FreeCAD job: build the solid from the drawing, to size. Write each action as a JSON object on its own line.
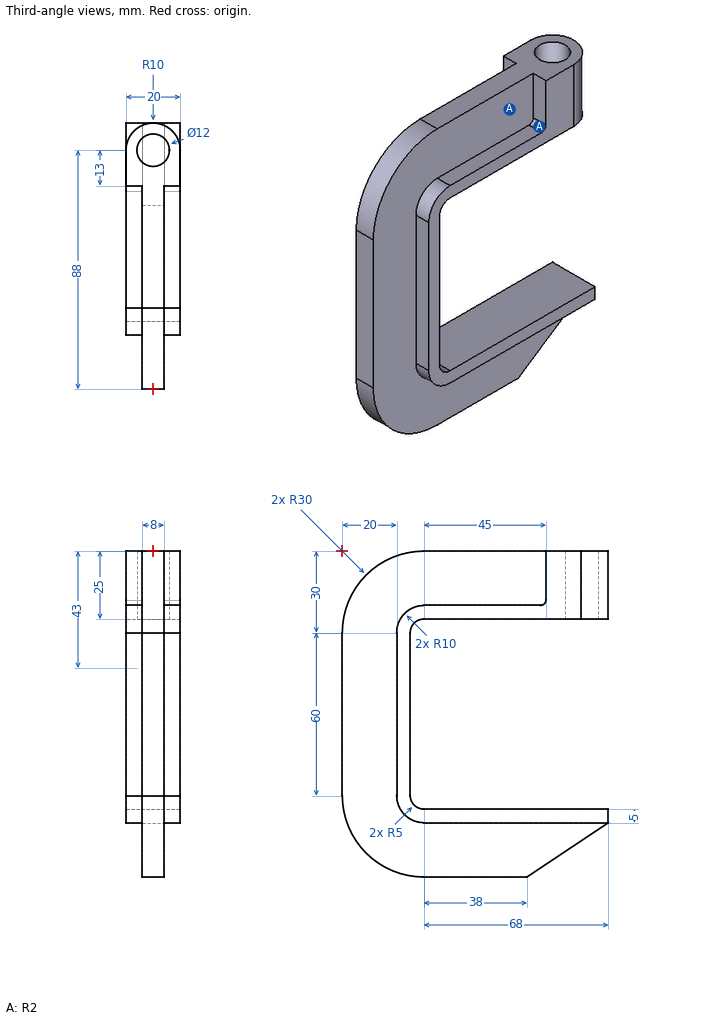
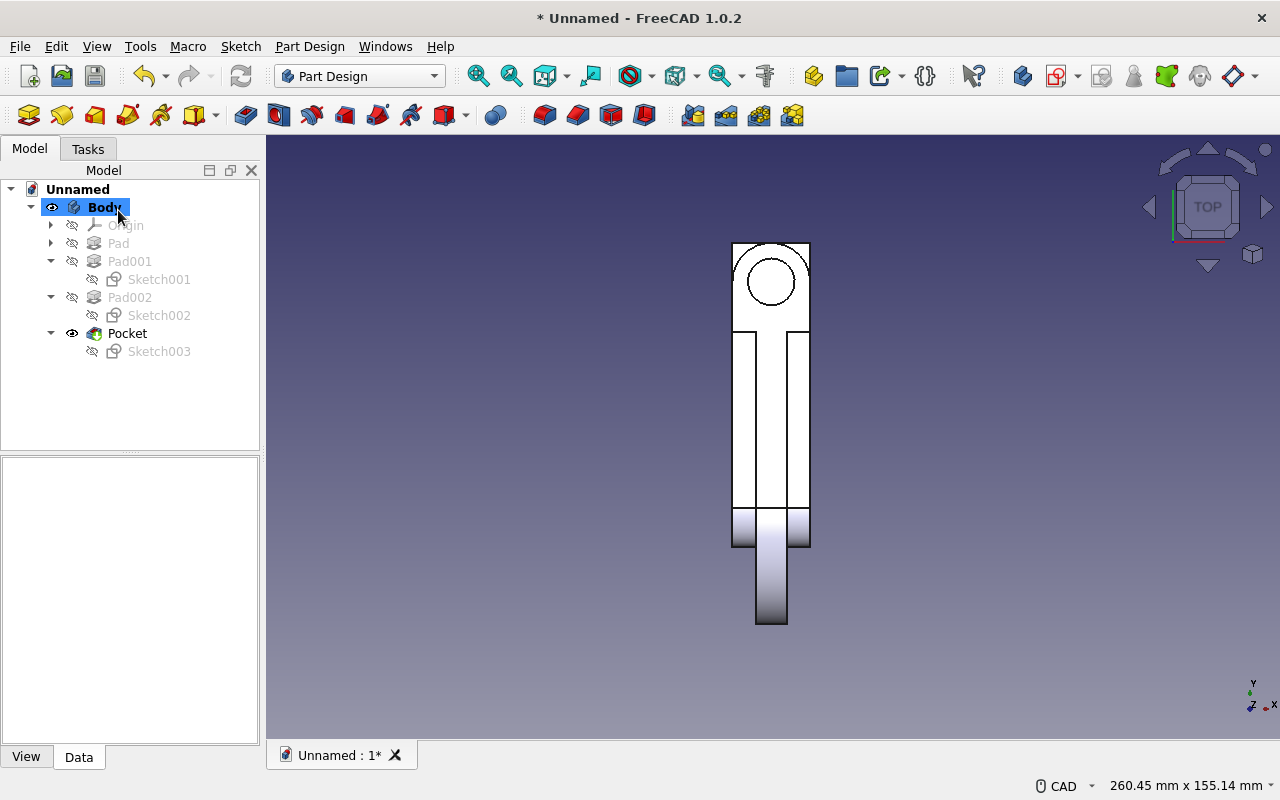
{"action": "key", "text": "1"}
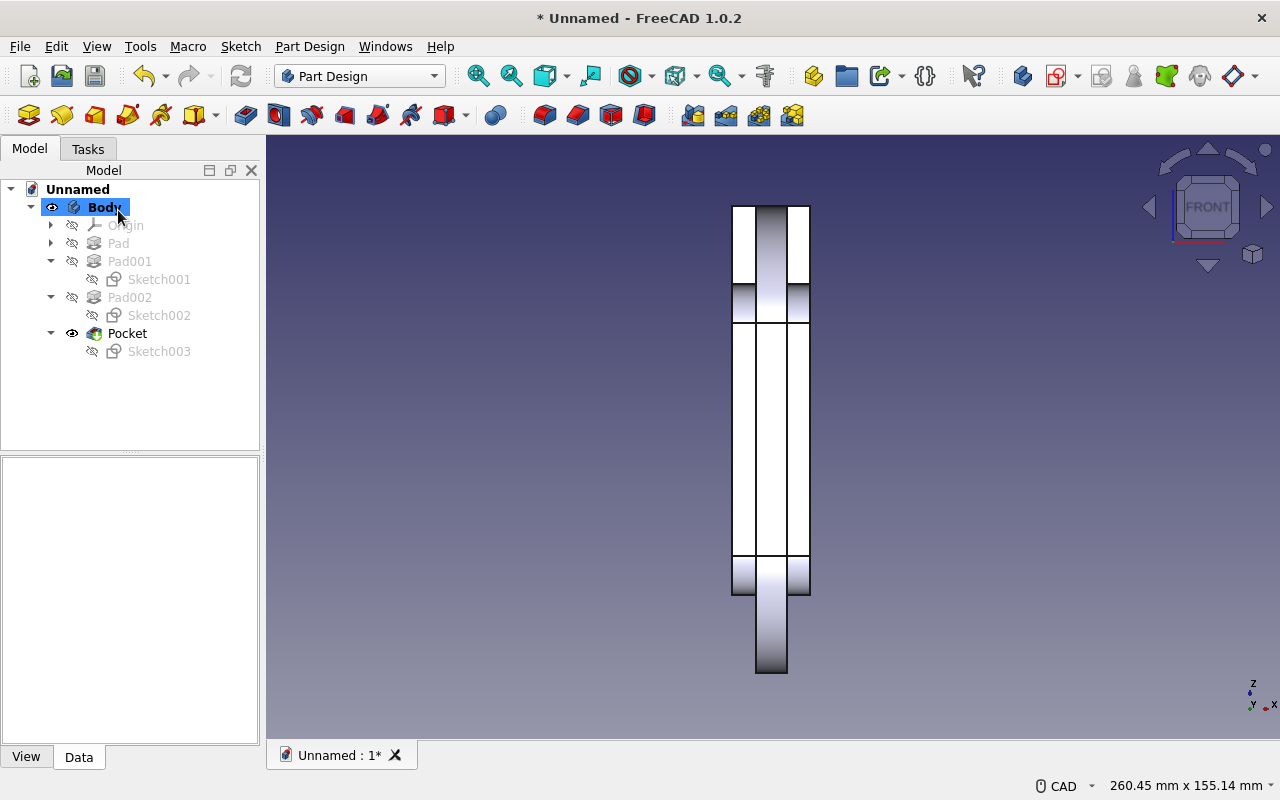
{"action": "key", "text": "3"}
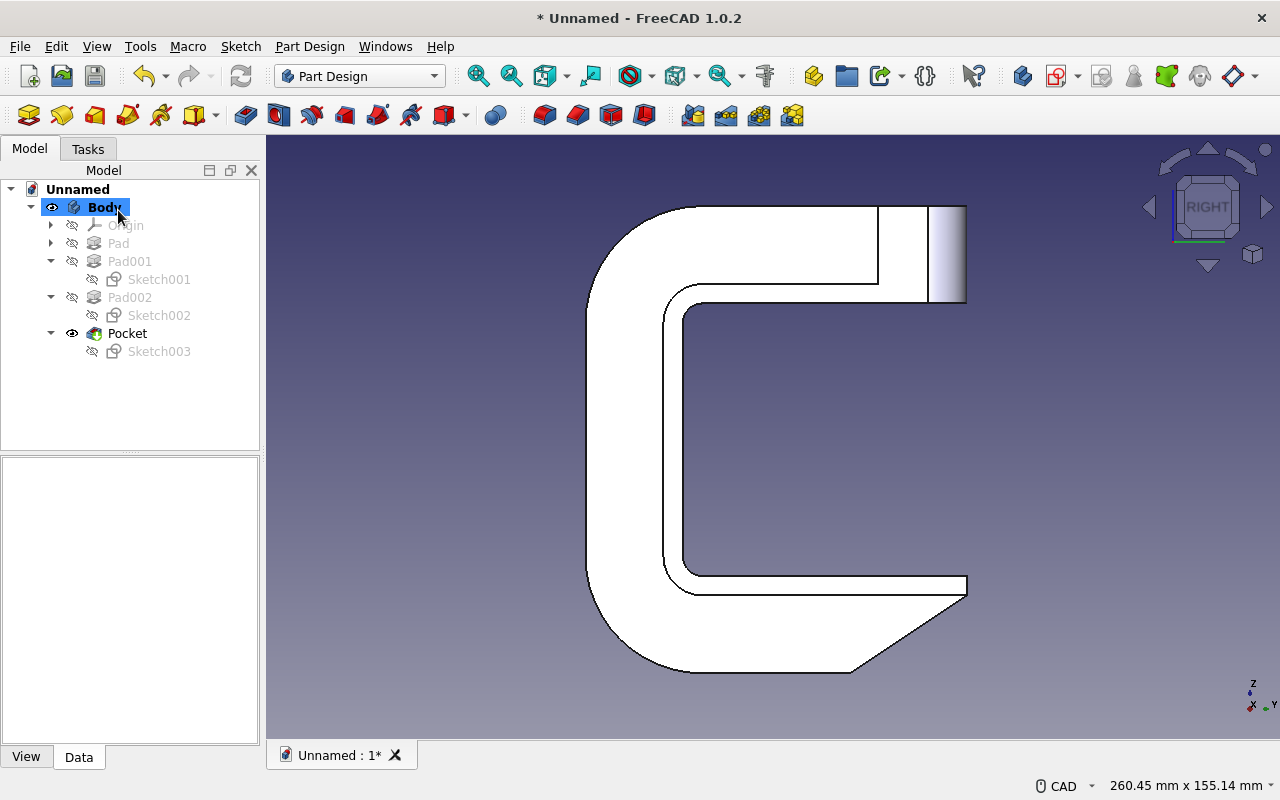
{"action": "key", "text": "5"}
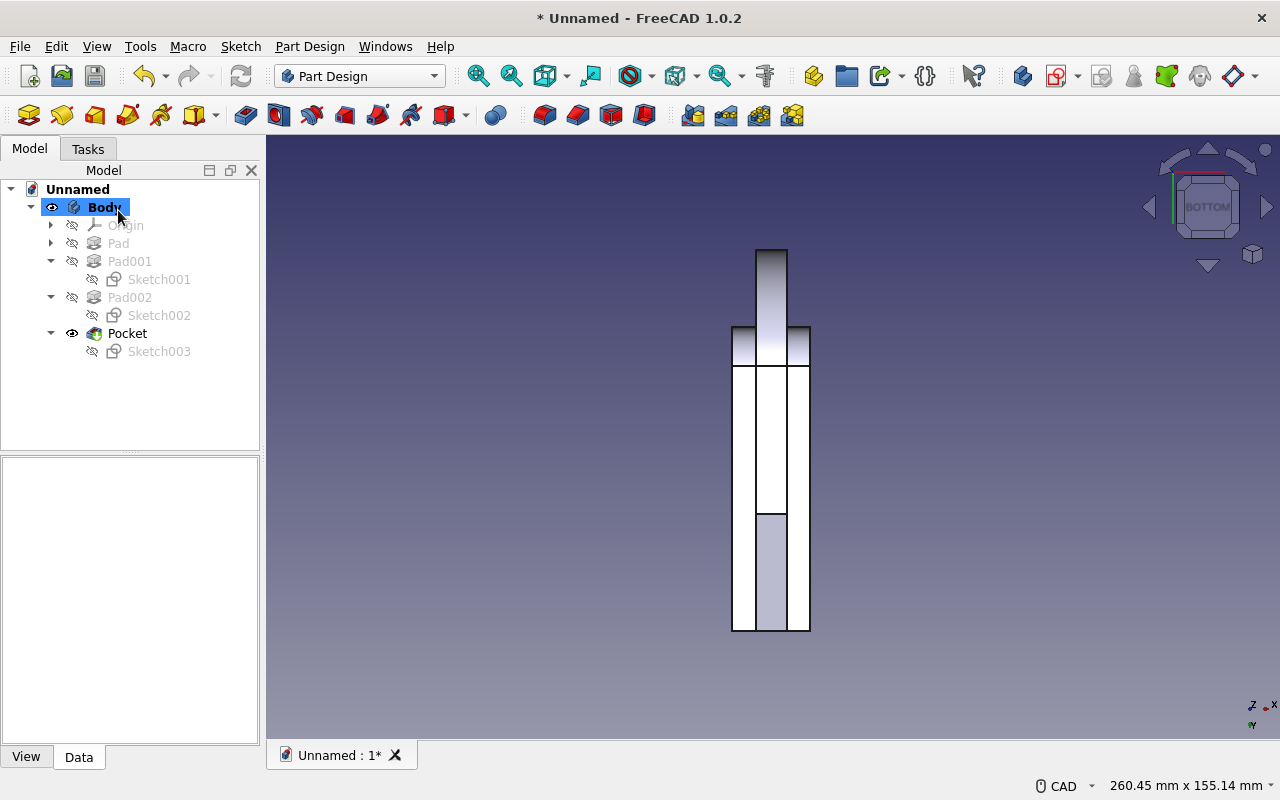
{"action": "key", "text": "4"}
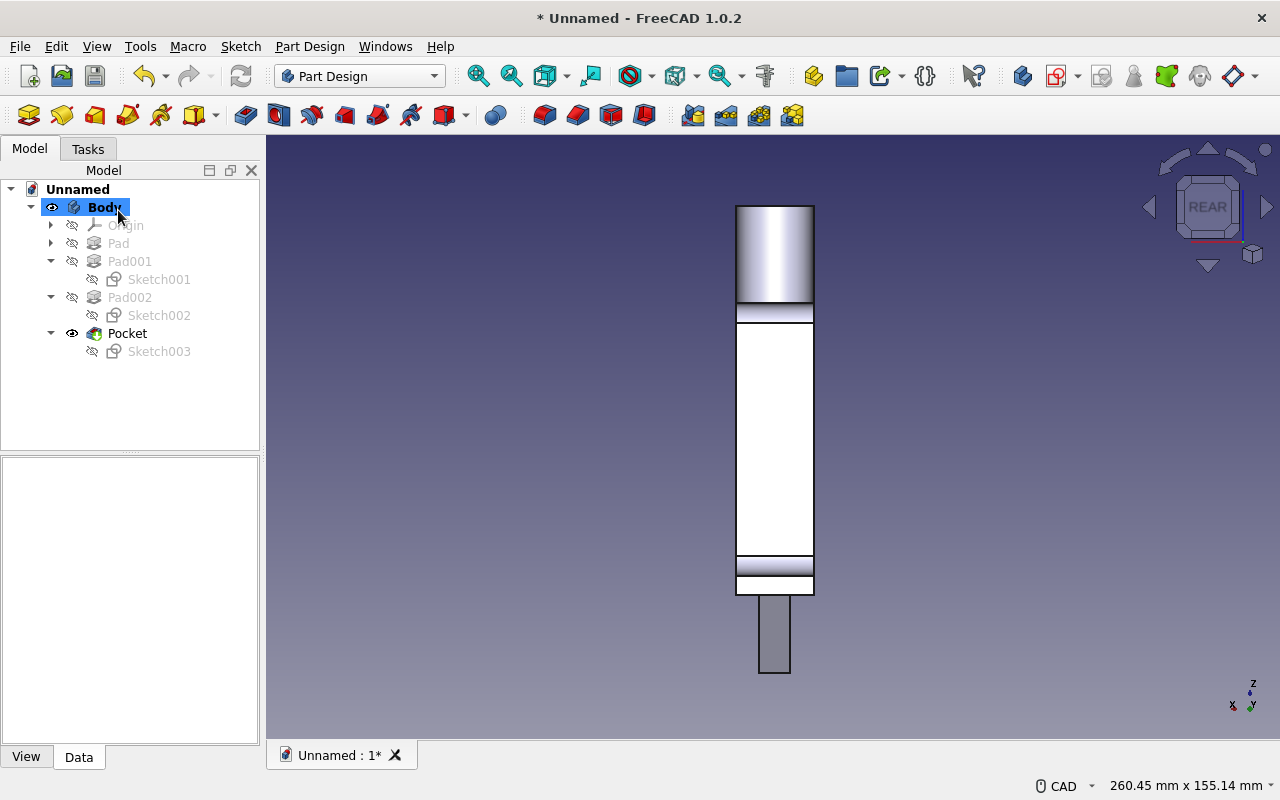
{"action": "key", "text": "6"}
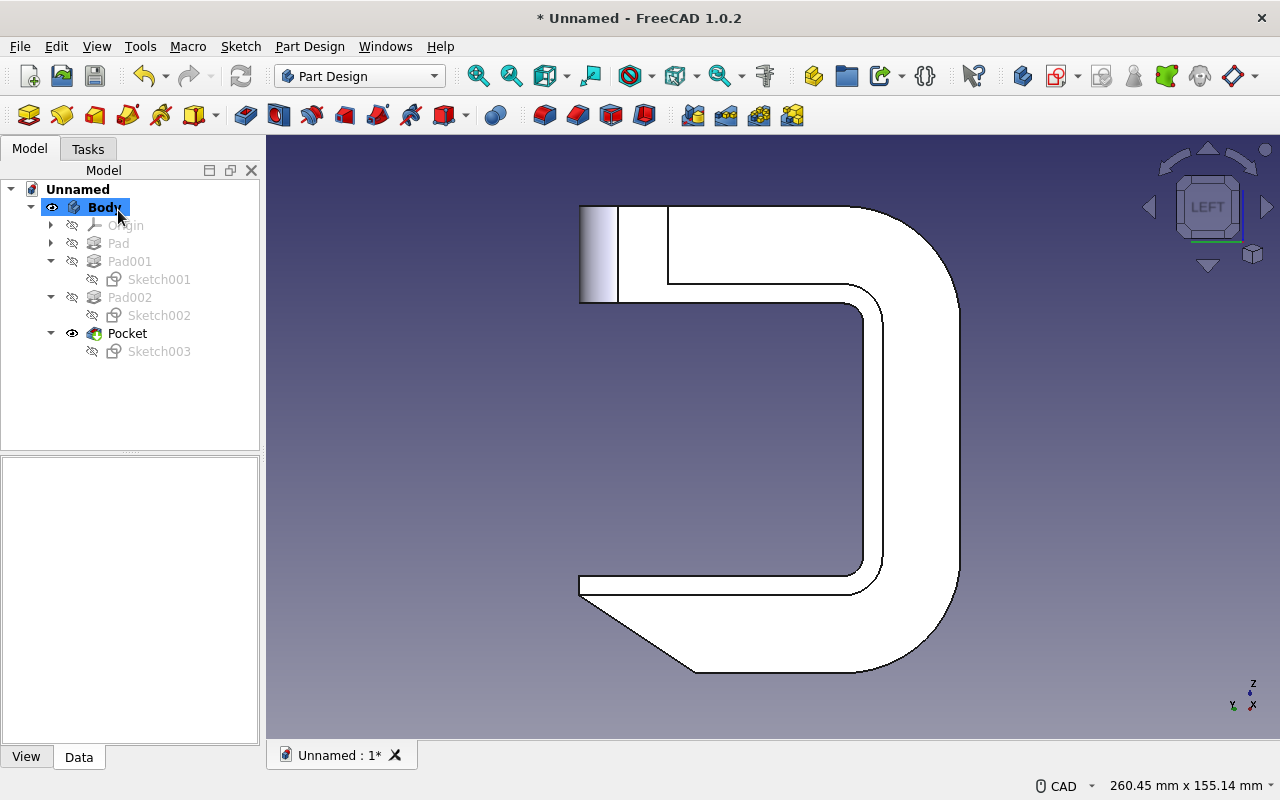
{"action": "key", "text": "v 3"}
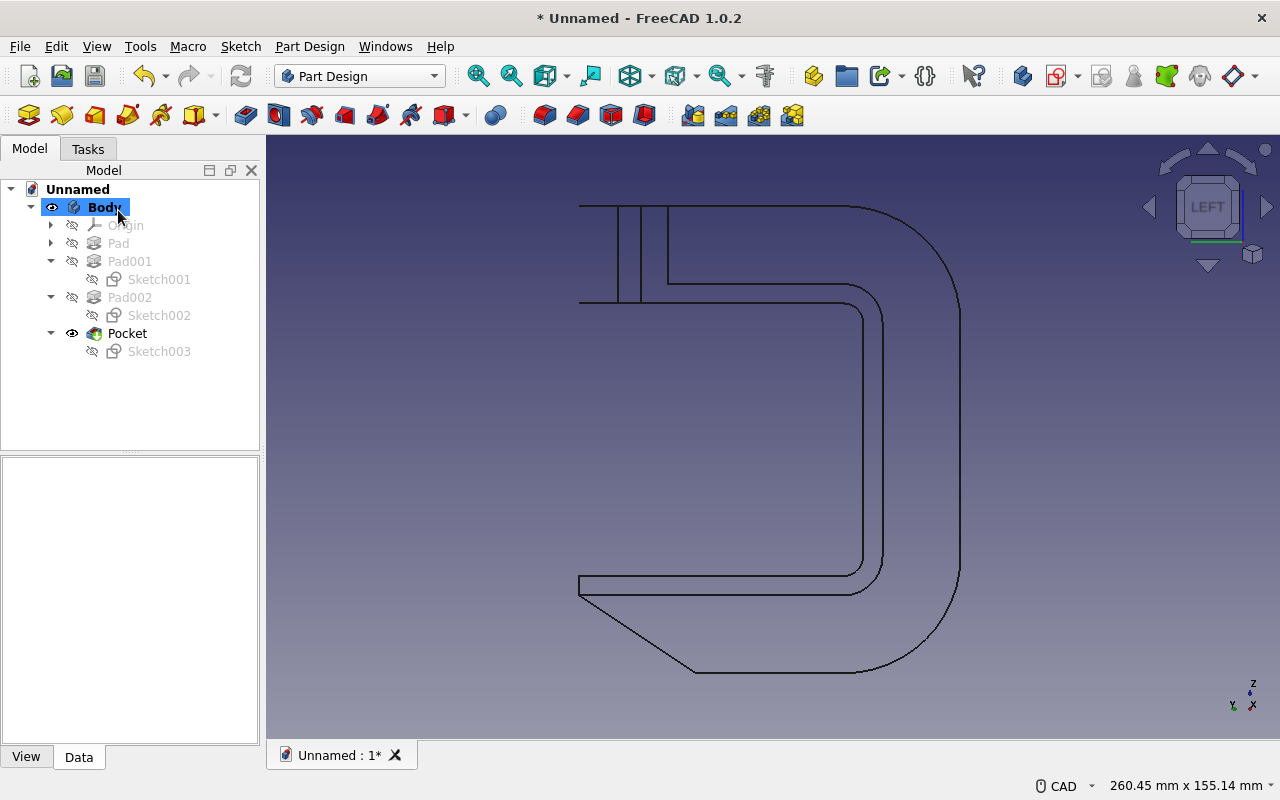
{"action": "key", "text": "0"}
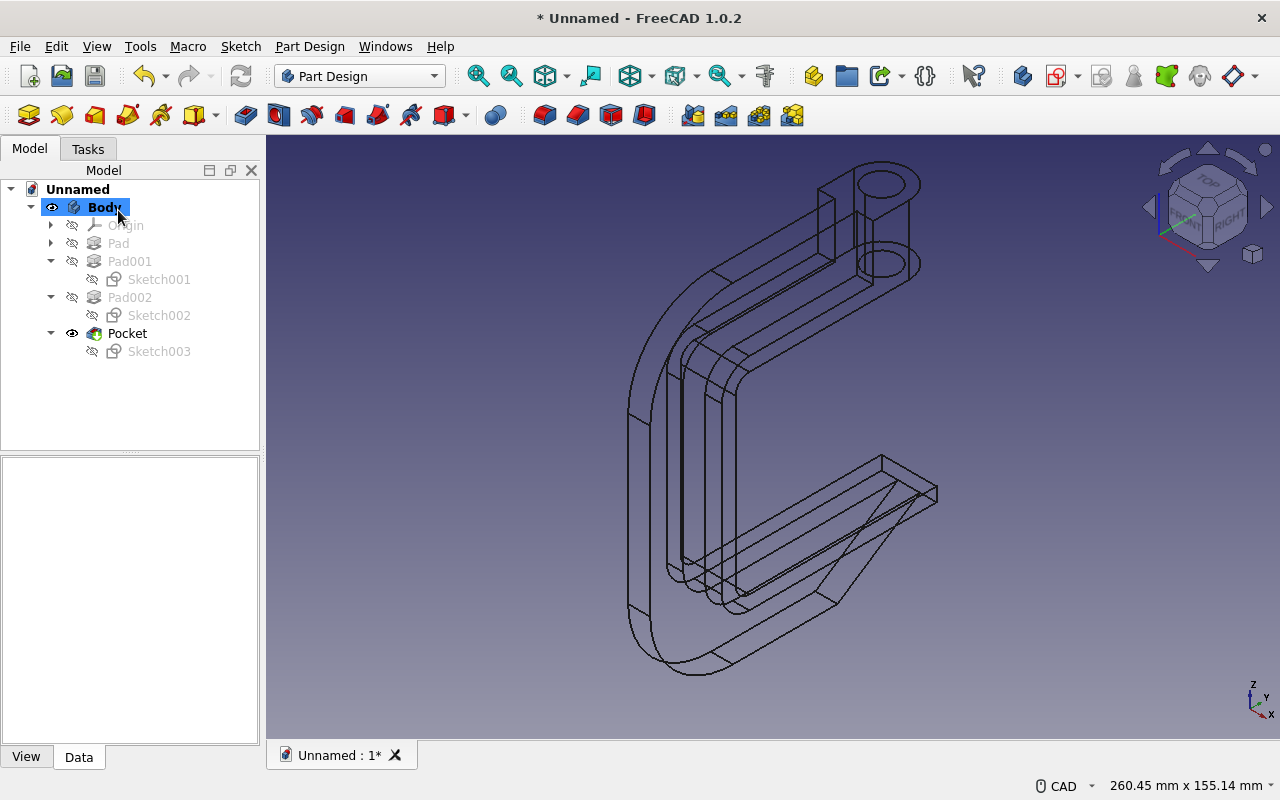
{"action": "left_click", "coordinate": [865, 279]}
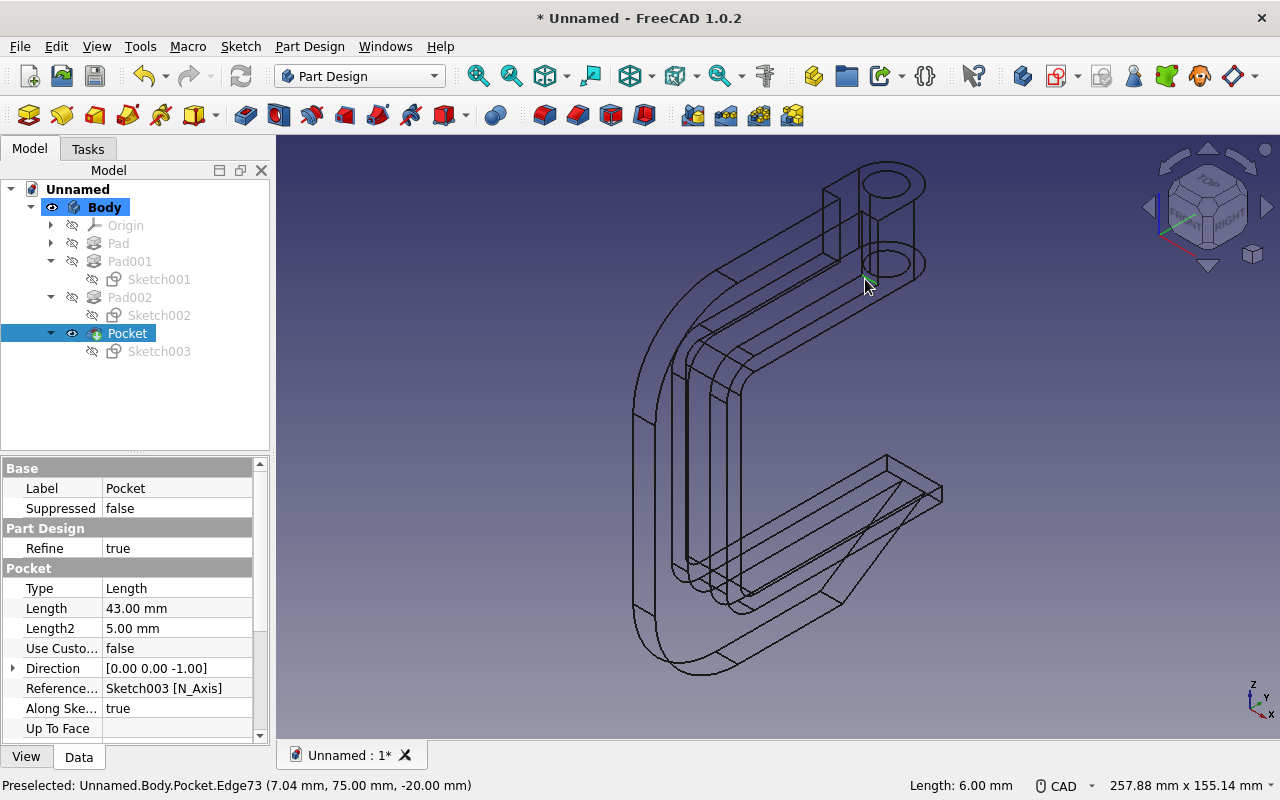
{"action": "left_click", "coordinate": [831, 257], "text": "ctrl"}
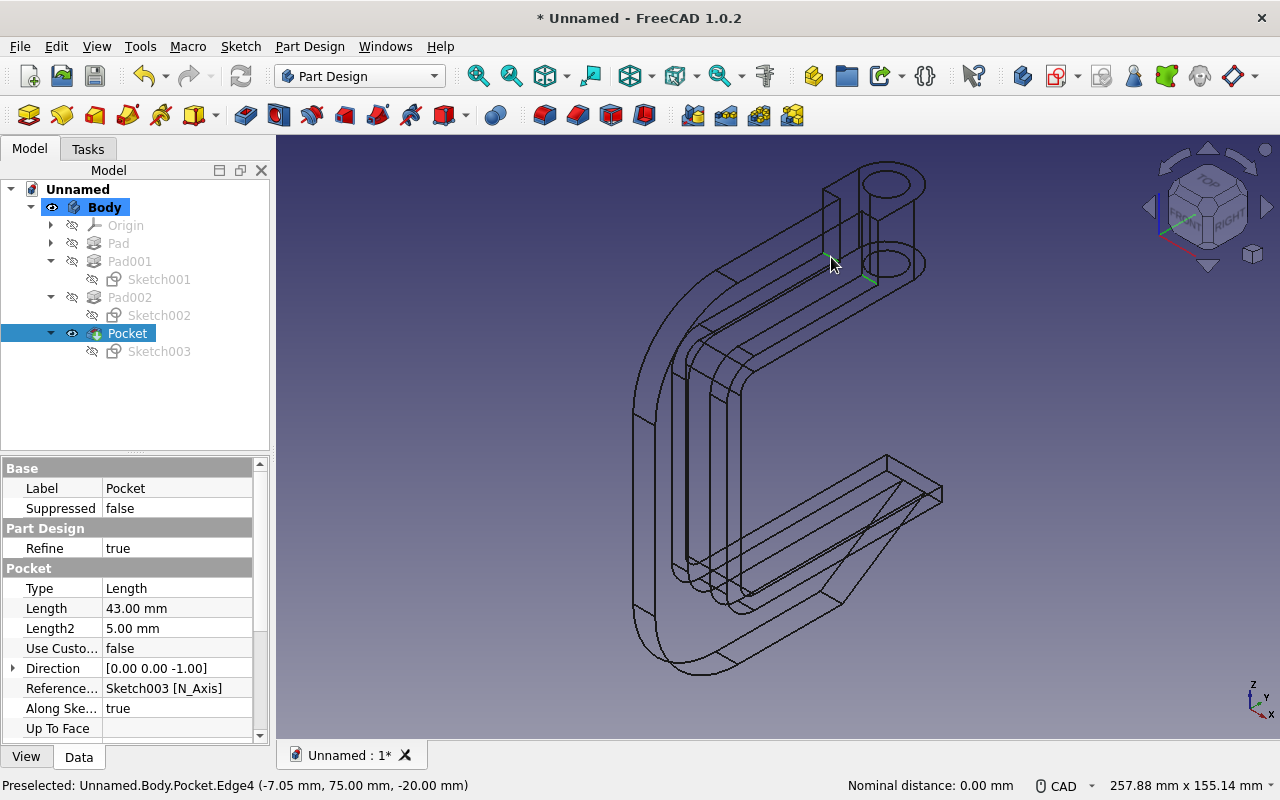
{"action": "key", "text": "v 1"}